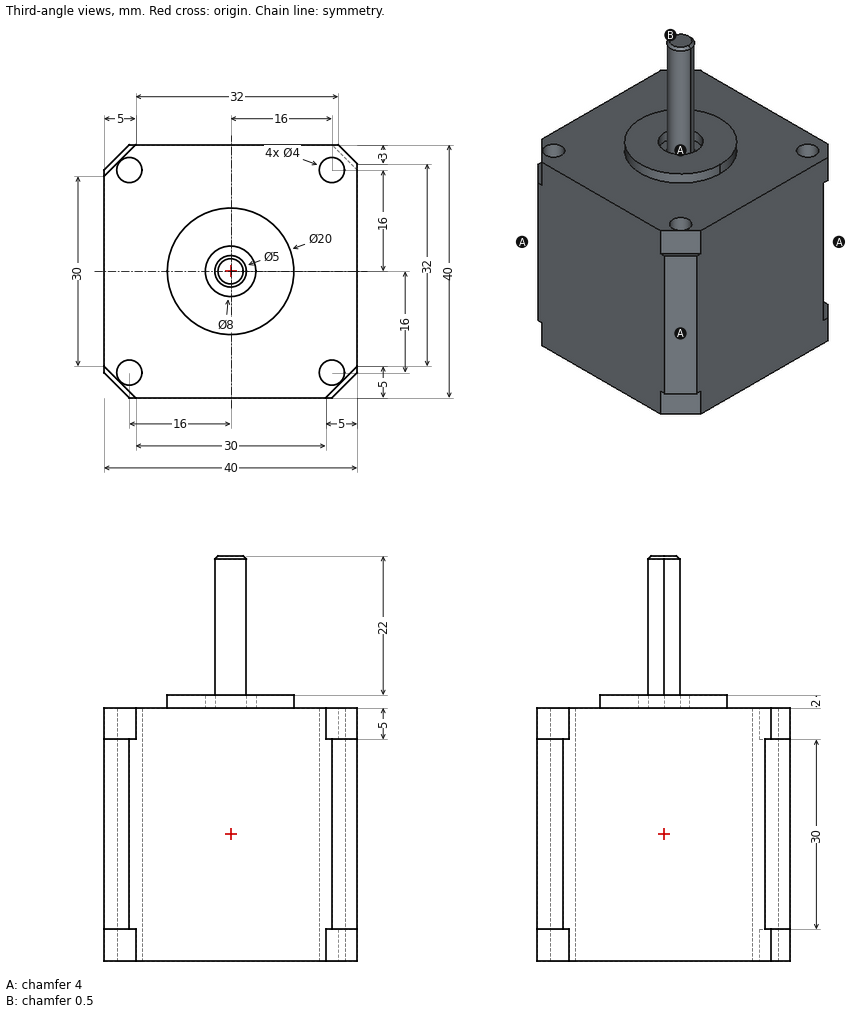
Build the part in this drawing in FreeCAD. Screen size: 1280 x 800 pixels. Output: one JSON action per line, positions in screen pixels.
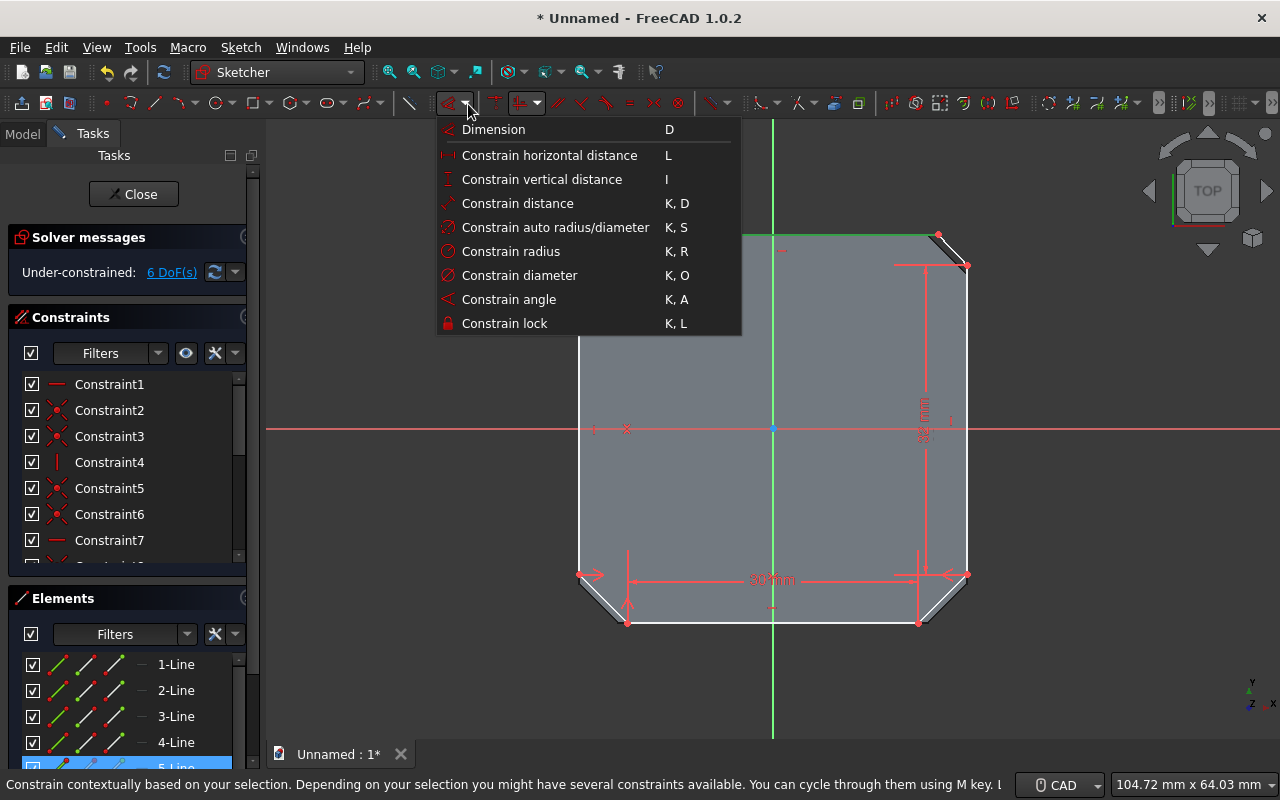
{"action": "left_click", "coordinate": [589, 155]}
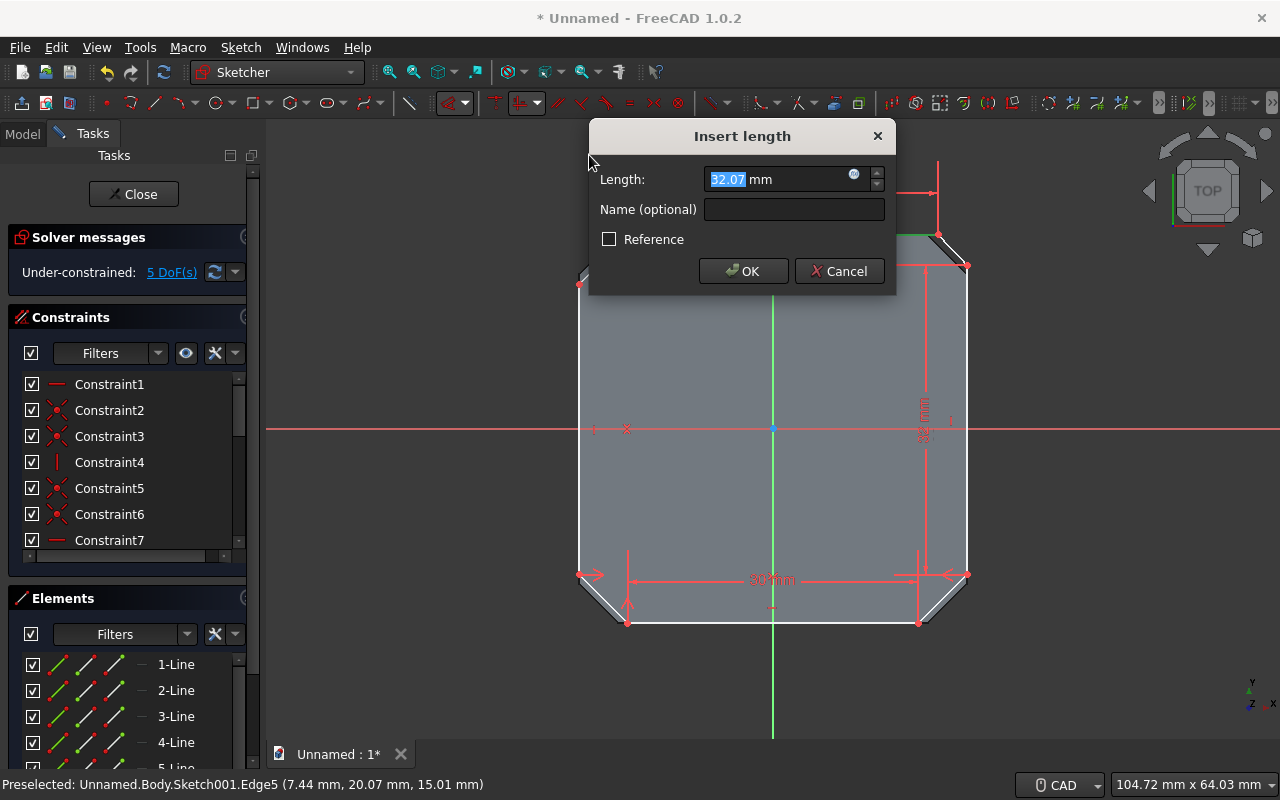
{"action": "type", "text": "32"}
{"action": "key", "text": "Return"}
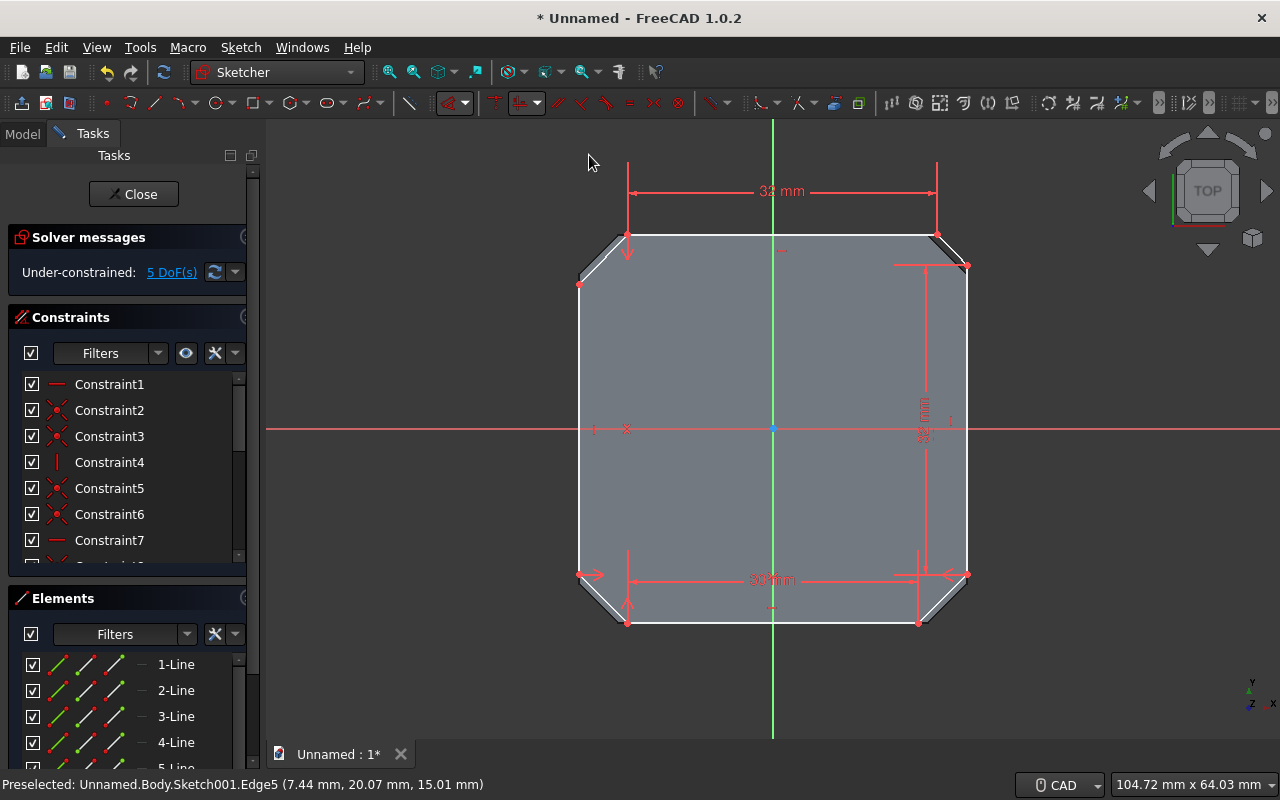
{"action": "left_click", "coordinate": [579, 372]}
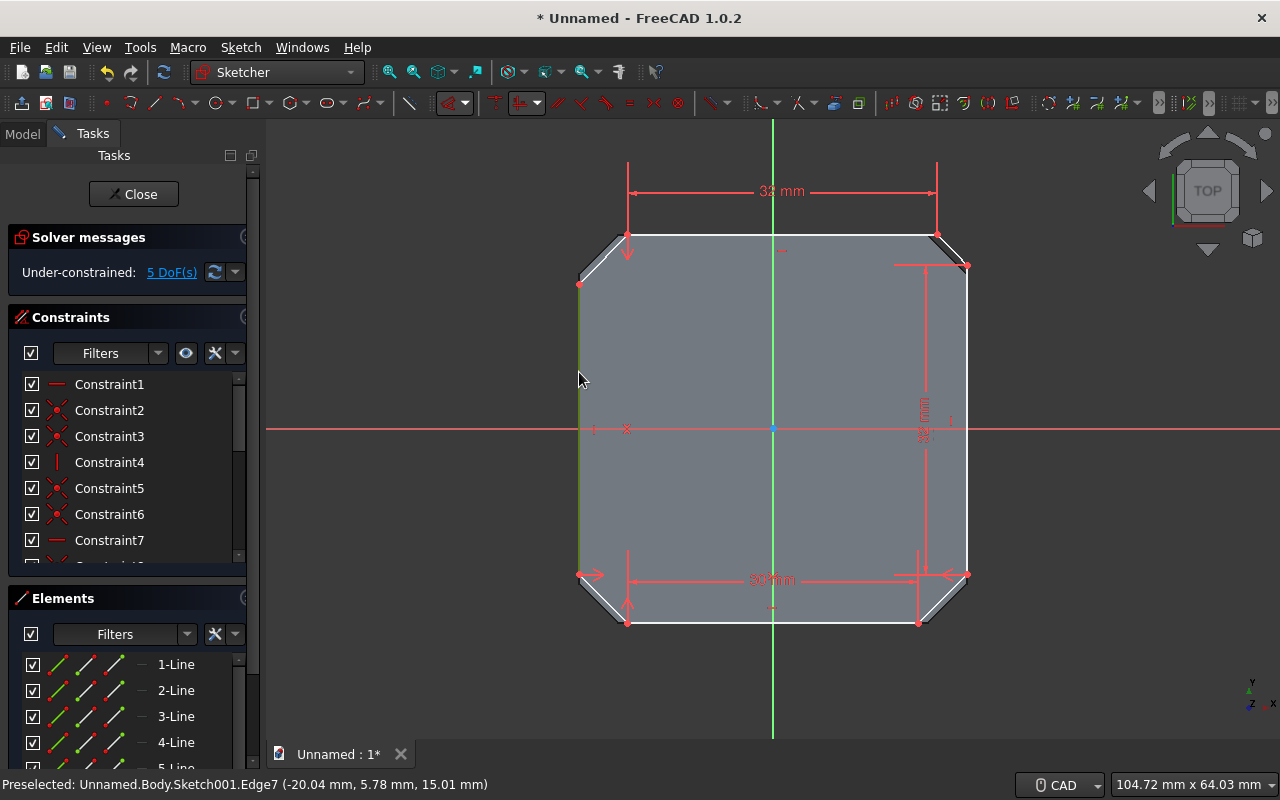
{"action": "key", "text": "i"}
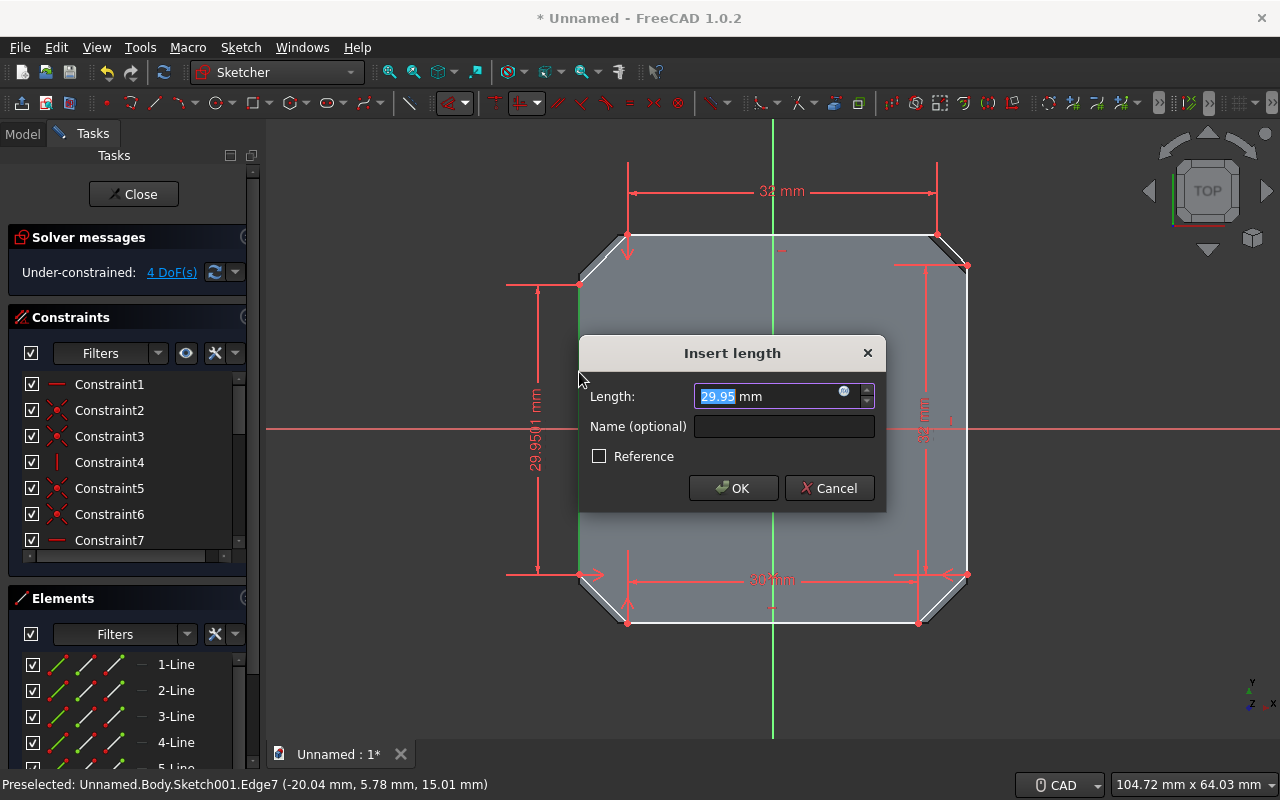
{"action": "type", "text": "30"}
{"action": "key", "text": "Return"}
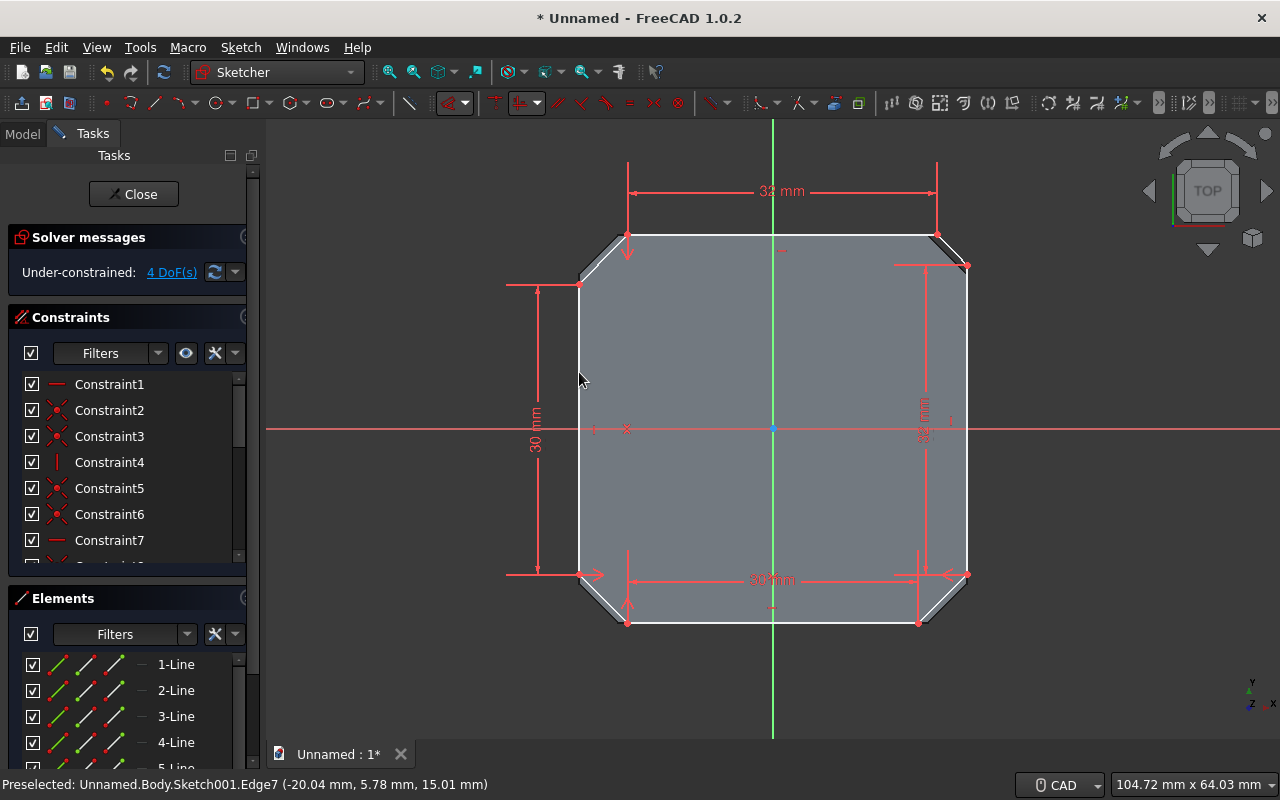
{"action": "left_click", "coordinate": [933, 609]}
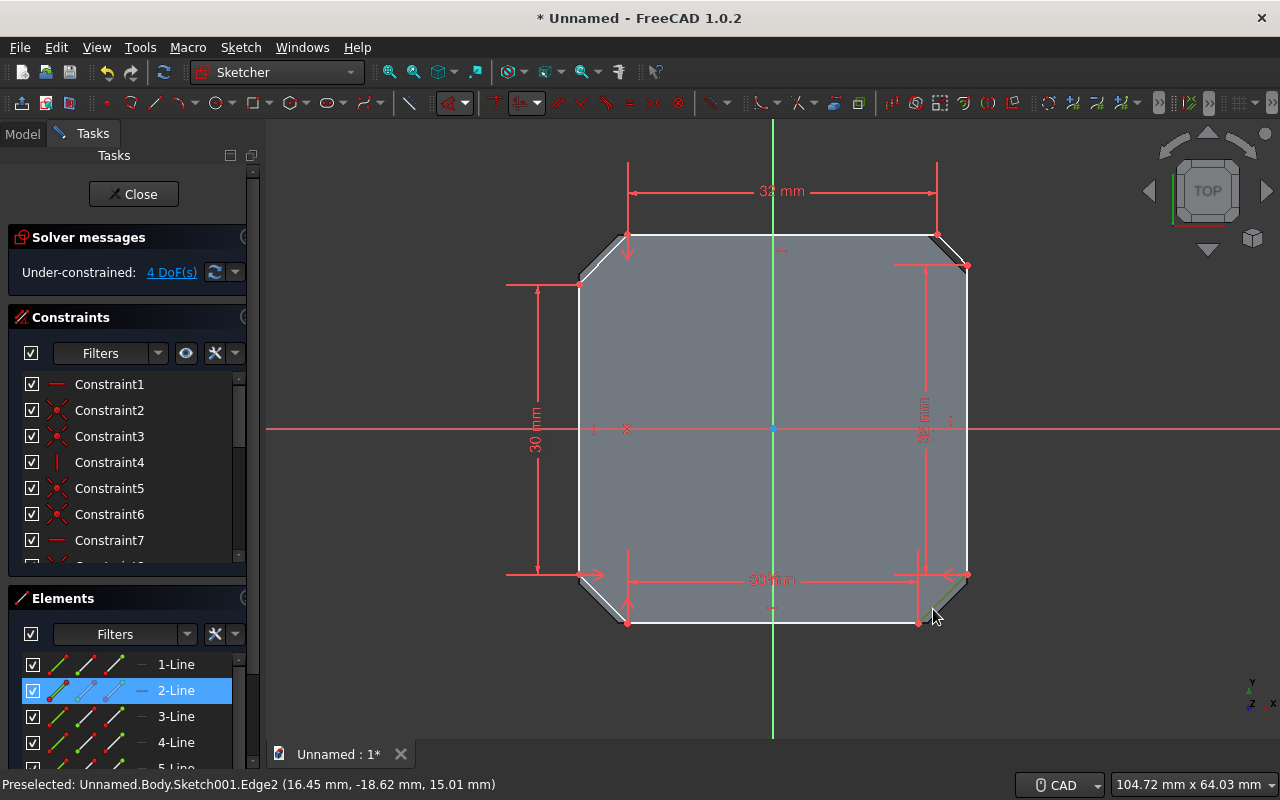
{"action": "key", "text": "l"}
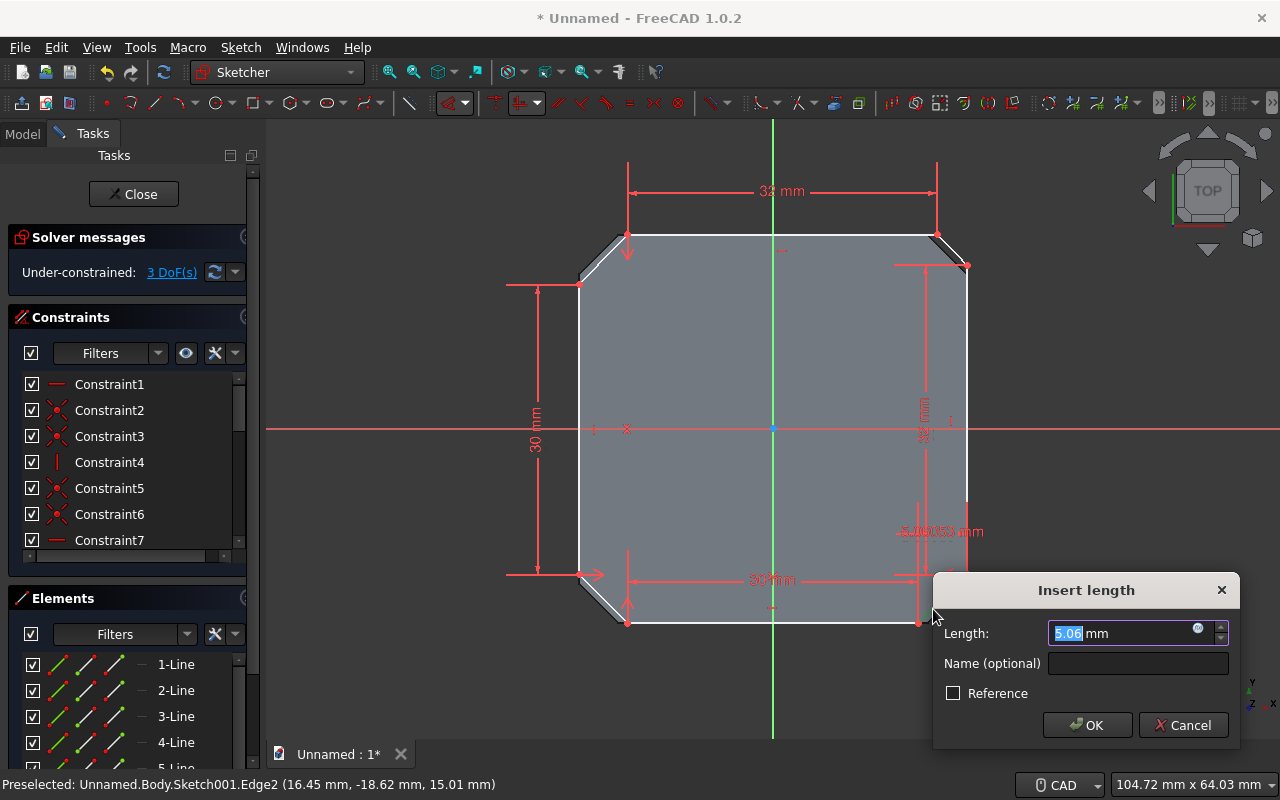
{"action": "type", "text": "5"}
{"action": "key", "text": "Return"}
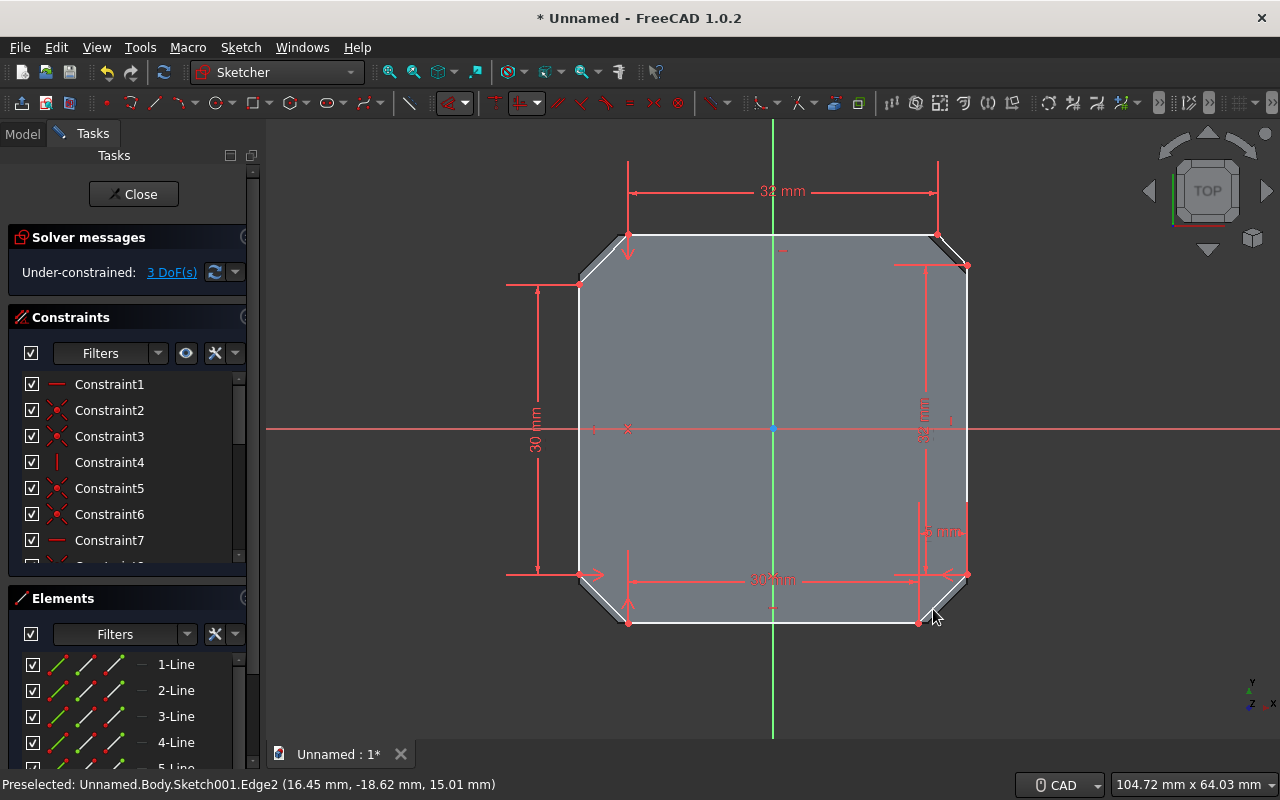
{"action": "left_click", "coordinate": [933, 609]}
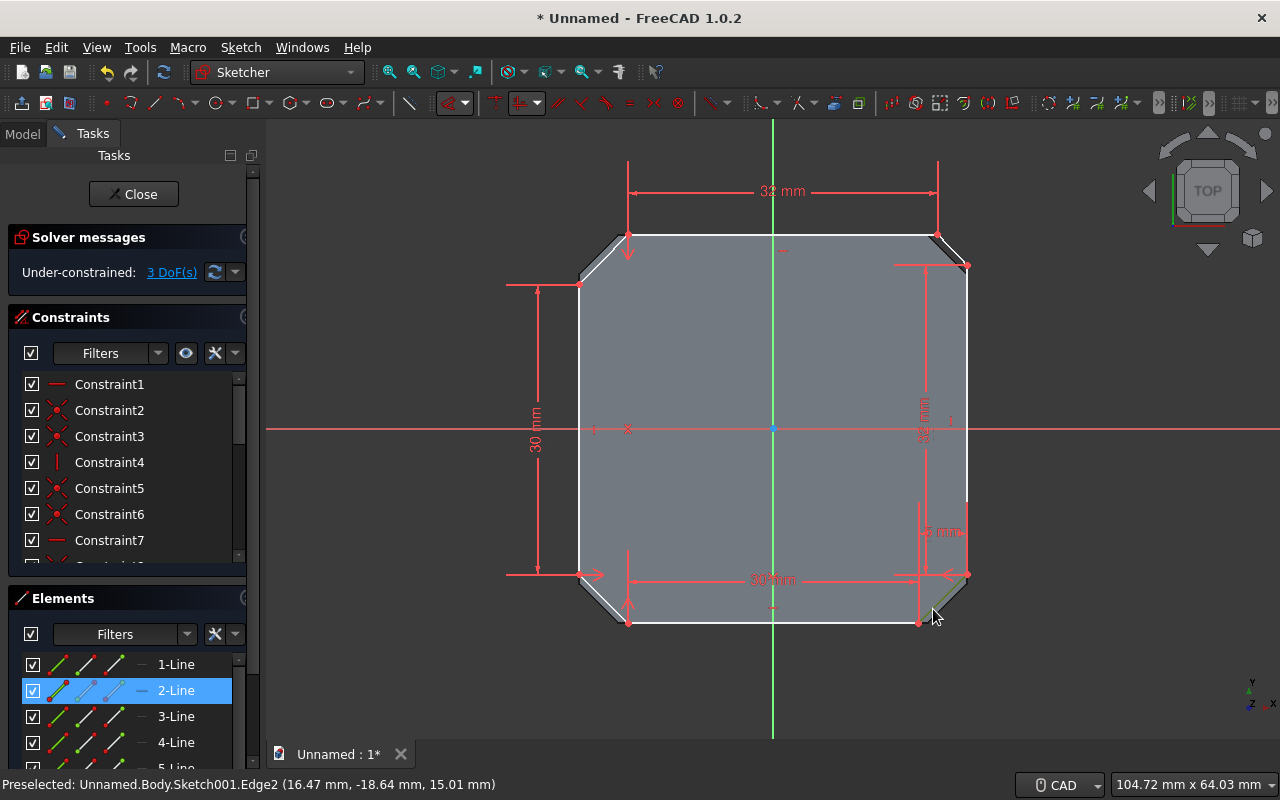
{"action": "left_click", "coordinate": [468, 104]}